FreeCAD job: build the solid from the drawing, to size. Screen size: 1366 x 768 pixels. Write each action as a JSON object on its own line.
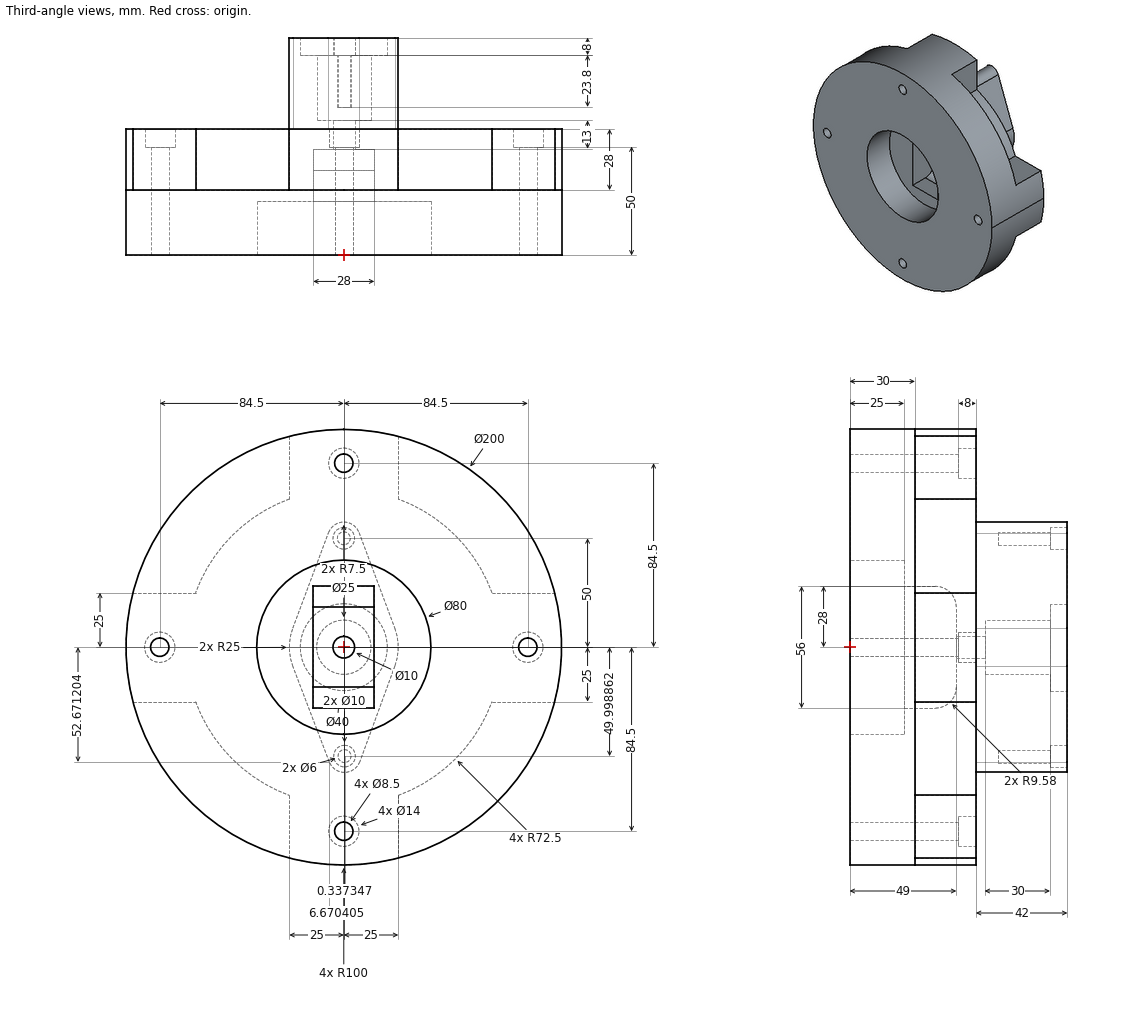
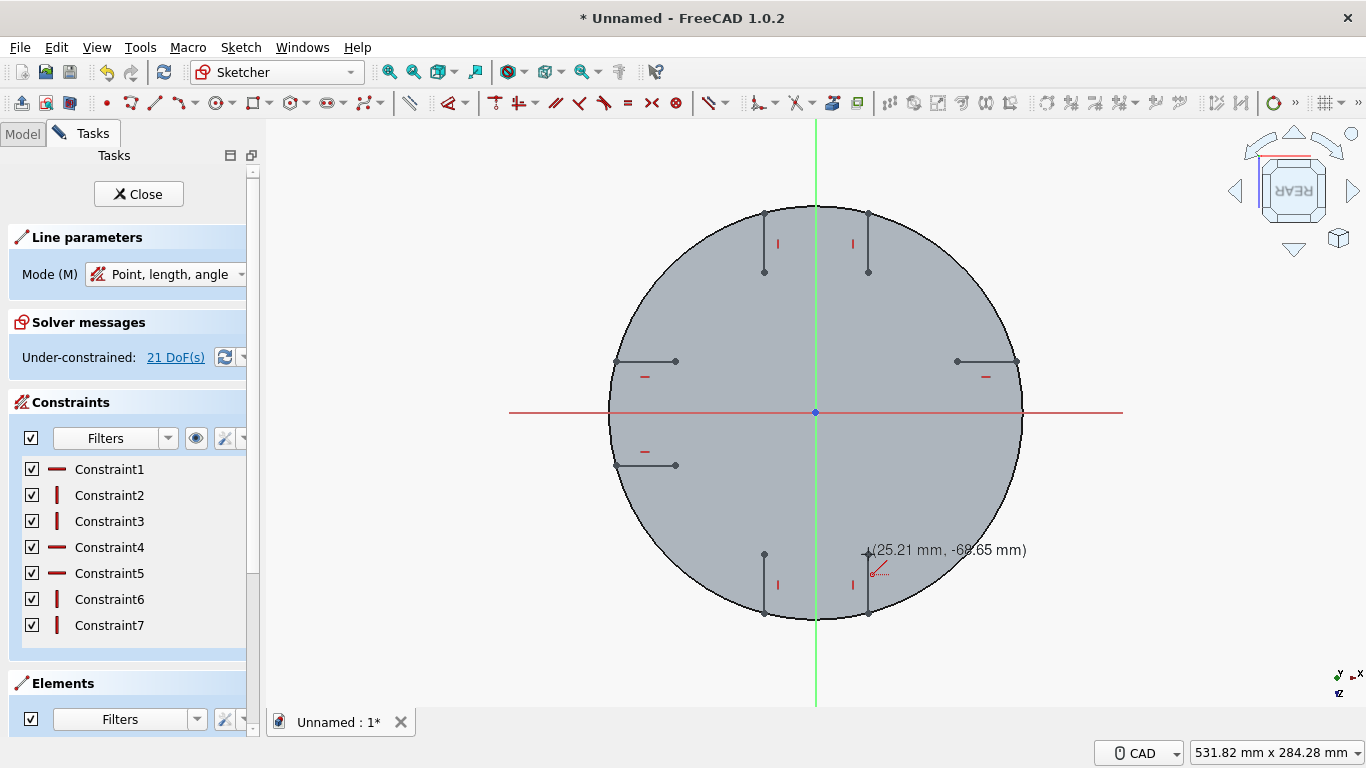
{"action": "left_click", "coordinate": [957, 465]}
{"action": "left_click", "coordinate": [1016, 465]}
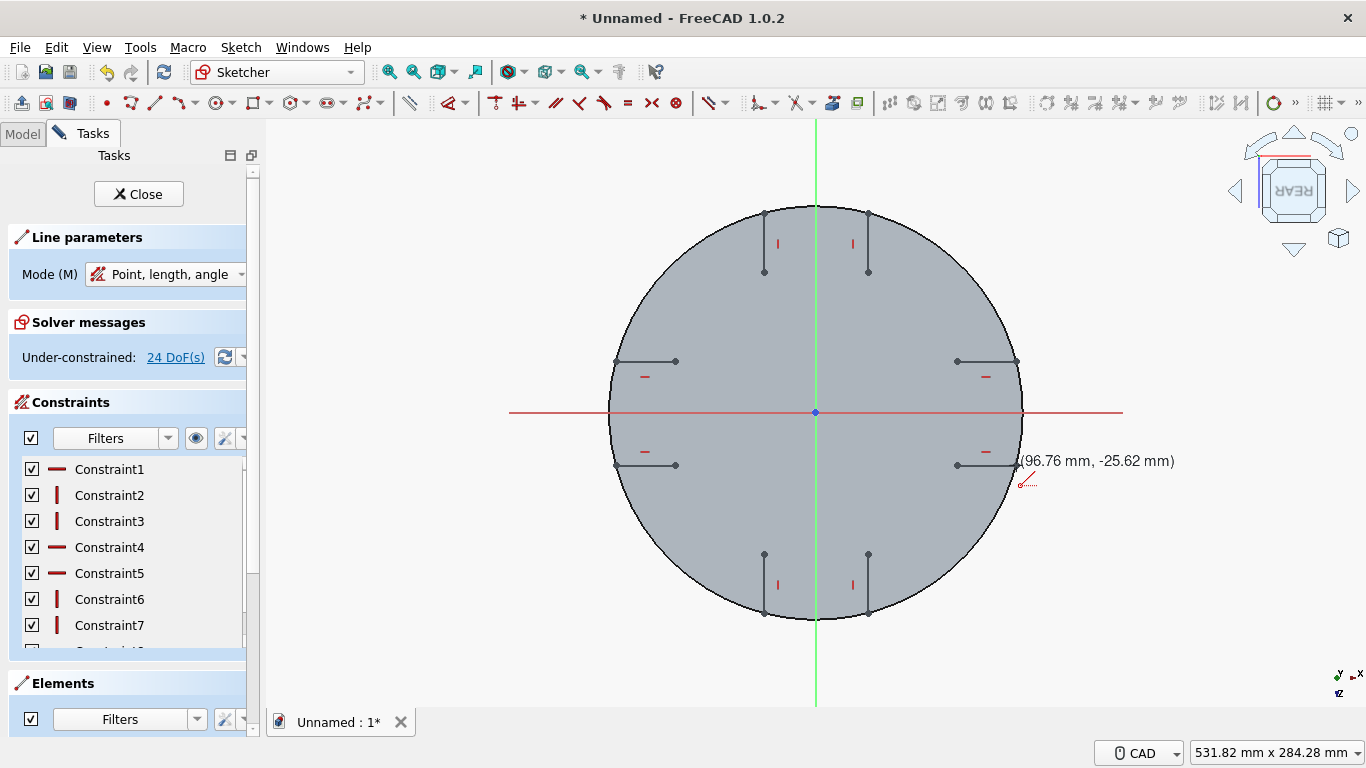
{"action": "left_click", "coordinate": [180, 104]}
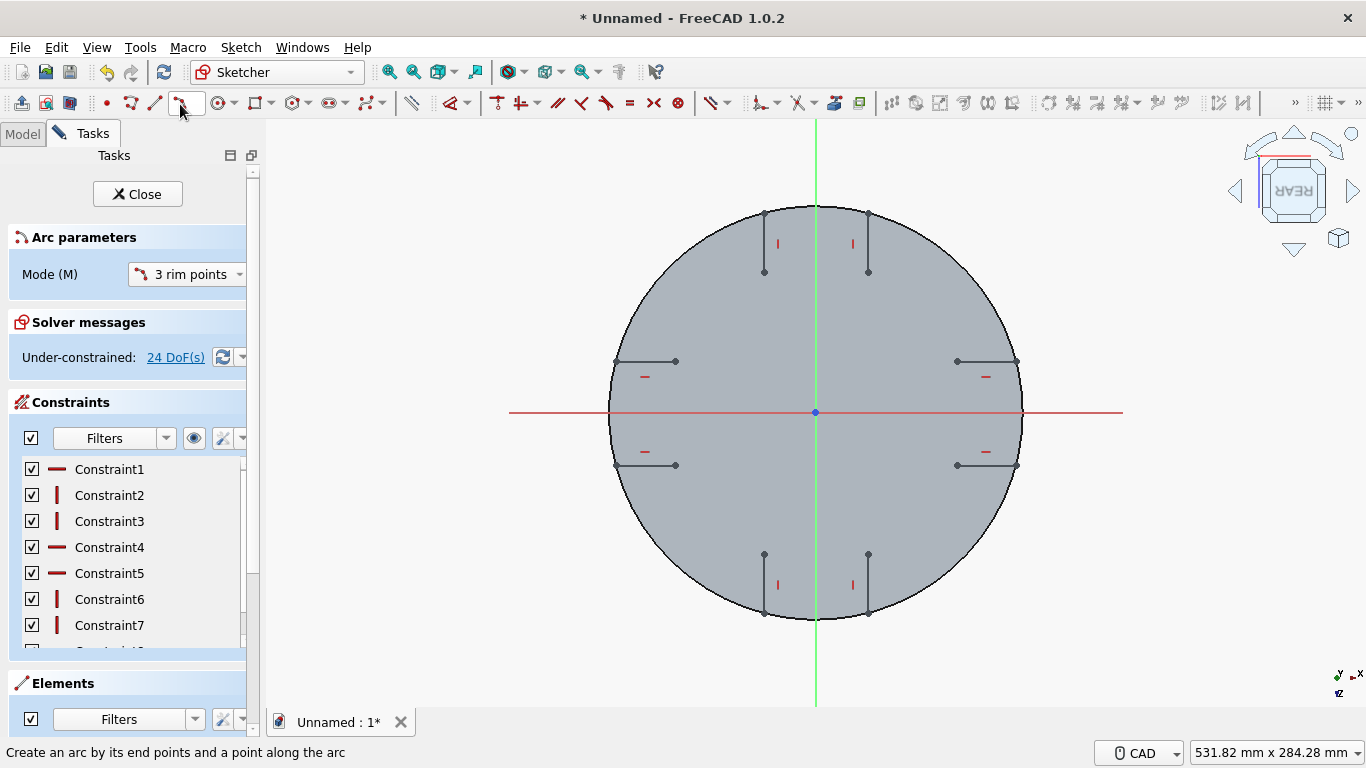
{"action": "left_click", "coordinate": [957, 362]}
{"action": "left_click", "coordinate": [868, 273]}
{"action": "left_click", "coordinate": [922, 307]}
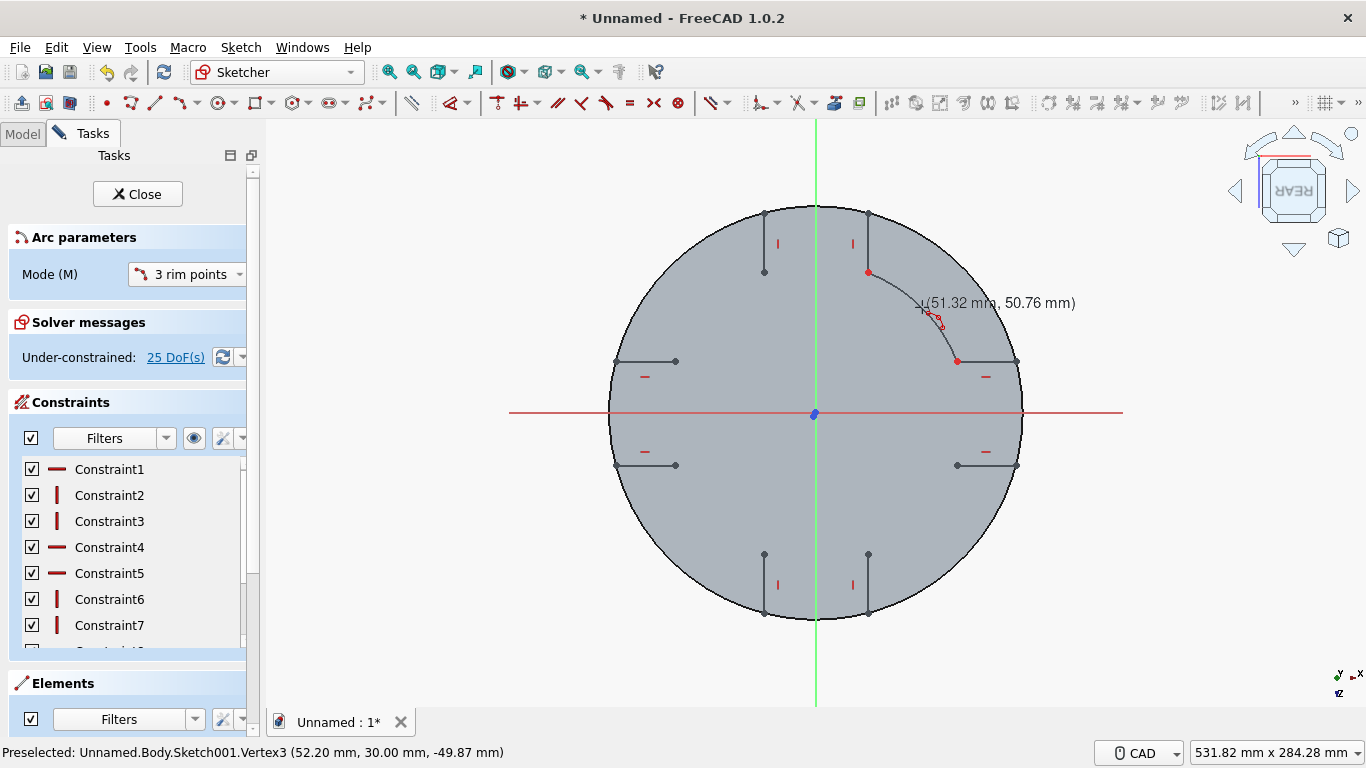
{"action": "left_click", "coordinate": [868, 214]}
{"action": "left_click", "coordinate": [764, 214]}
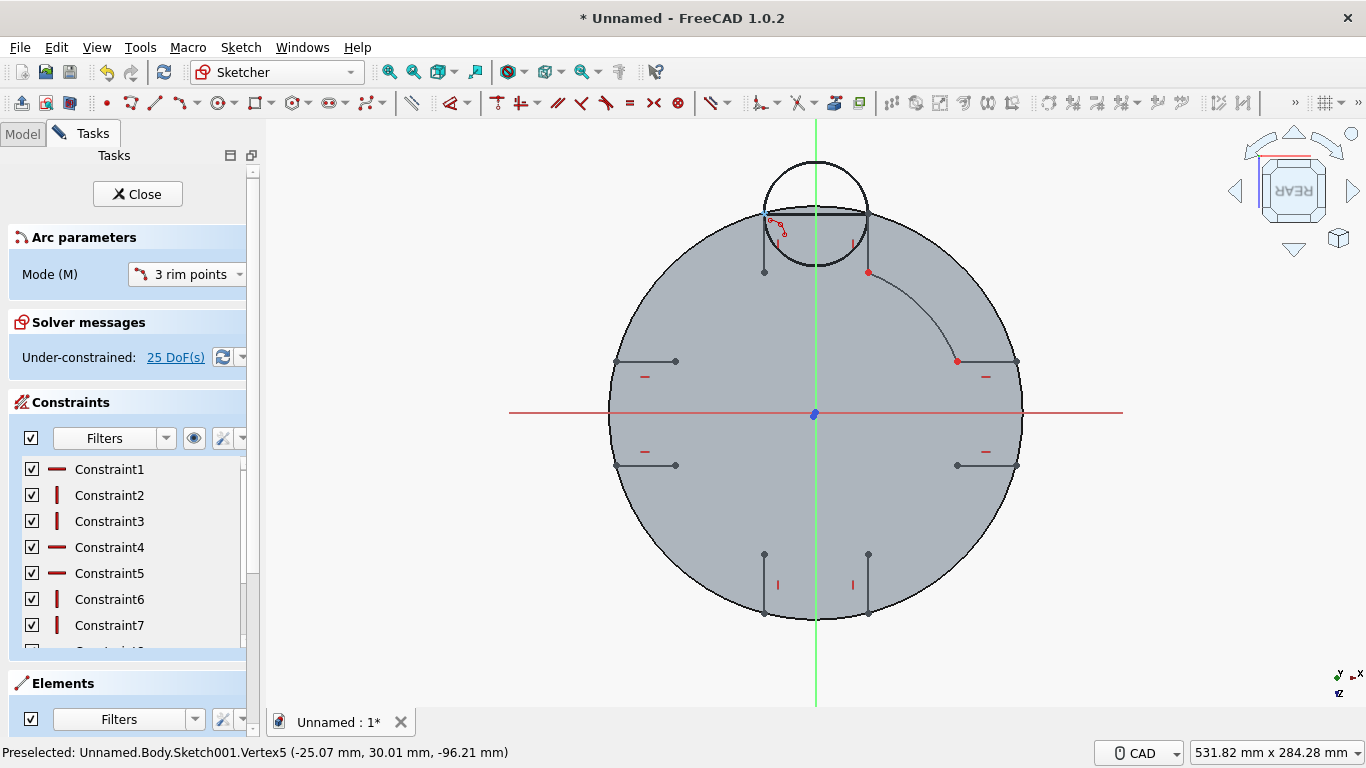
{"action": "scroll", "coordinate": [826, 206], "scroll_direction": "up", "scroll_amount": 5}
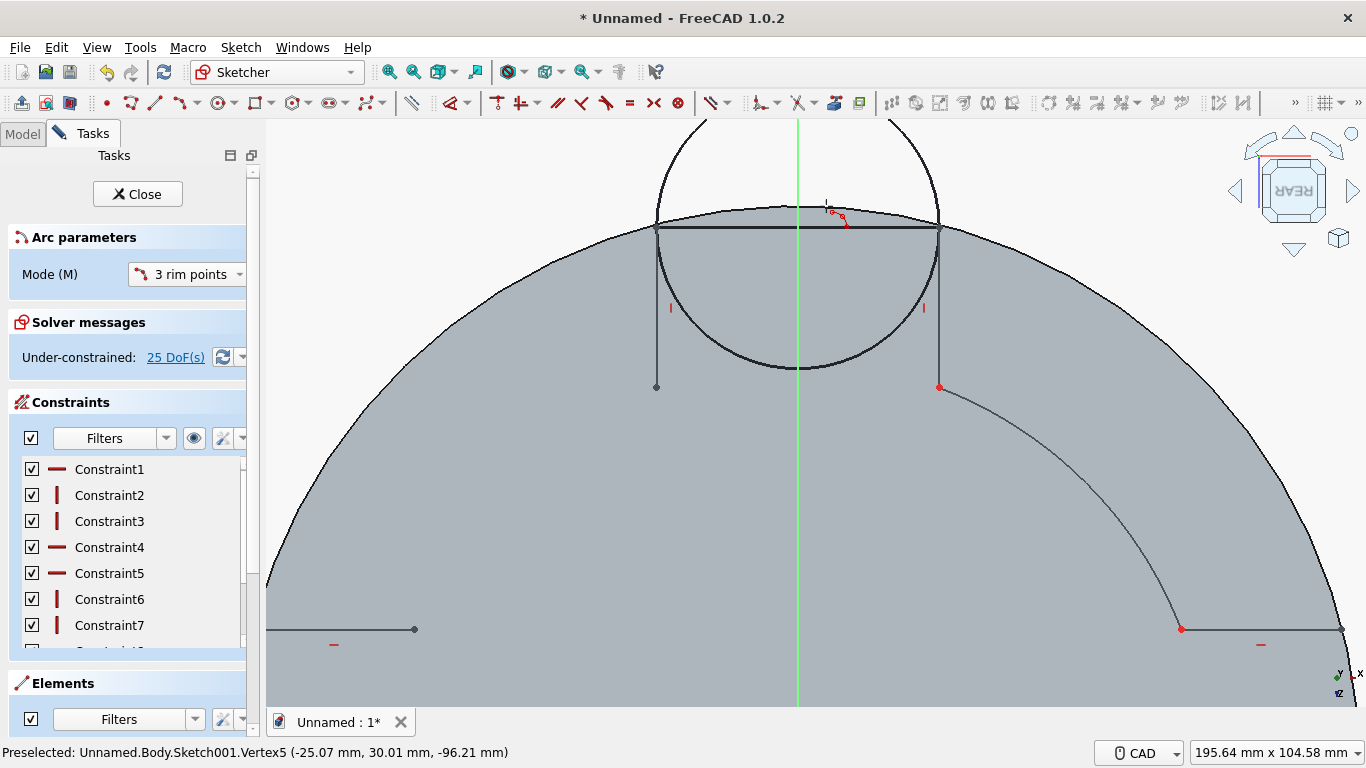
{"action": "left_click", "coordinate": [826, 207]}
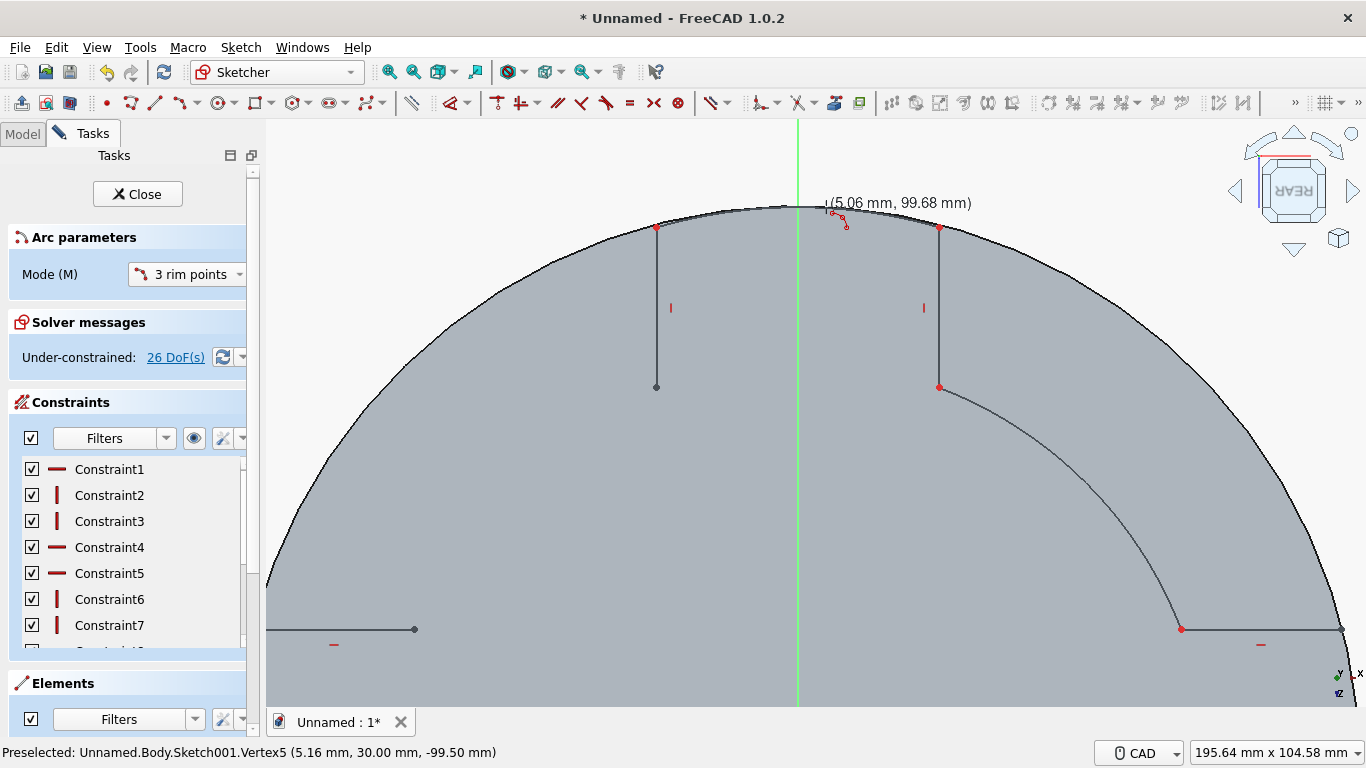
{"action": "left_click", "coordinate": [657, 388]}
{"action": "left_click", "coordinate": [415, 630]}
{"action": "left_click", "coordinate": [509, 480]}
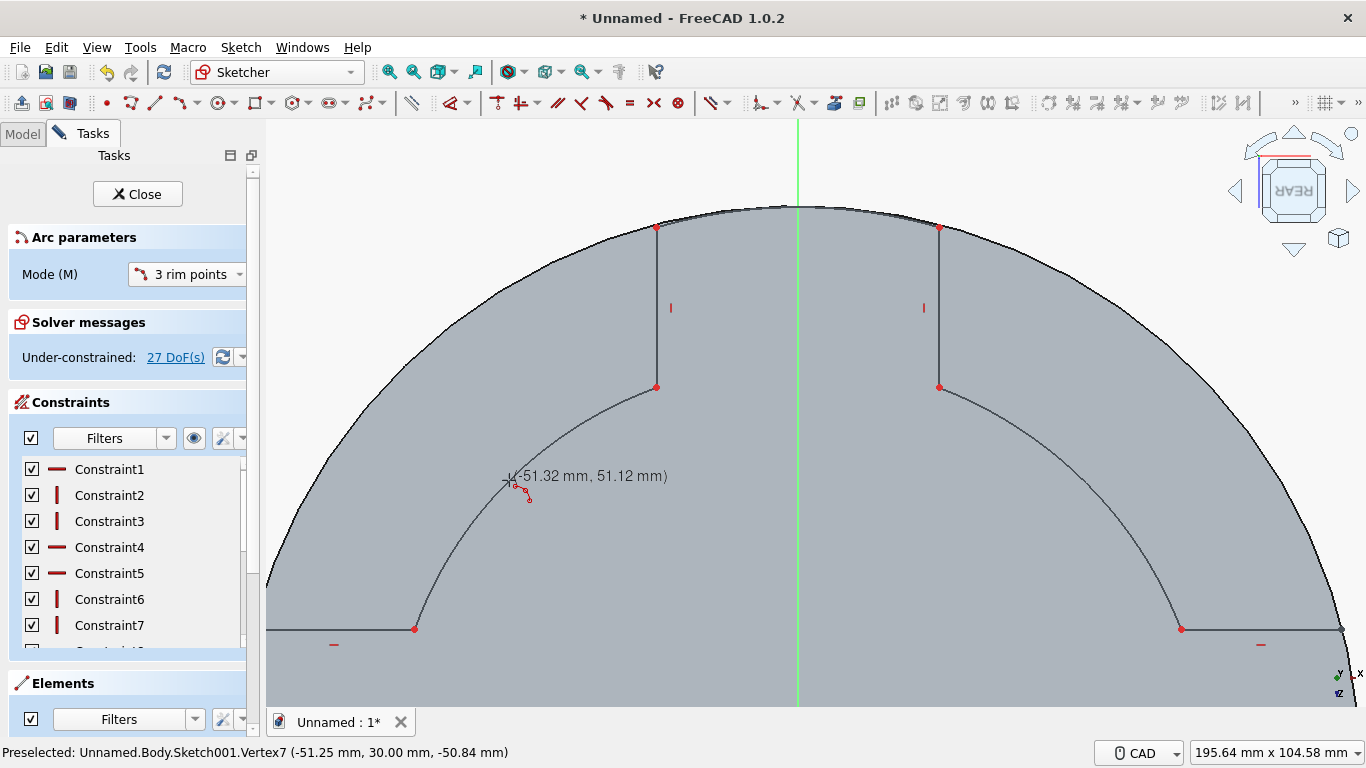
{"action": "scroll", "coordinate": [718, 206], "scroll_direction": "down", "scroll_amount": 5}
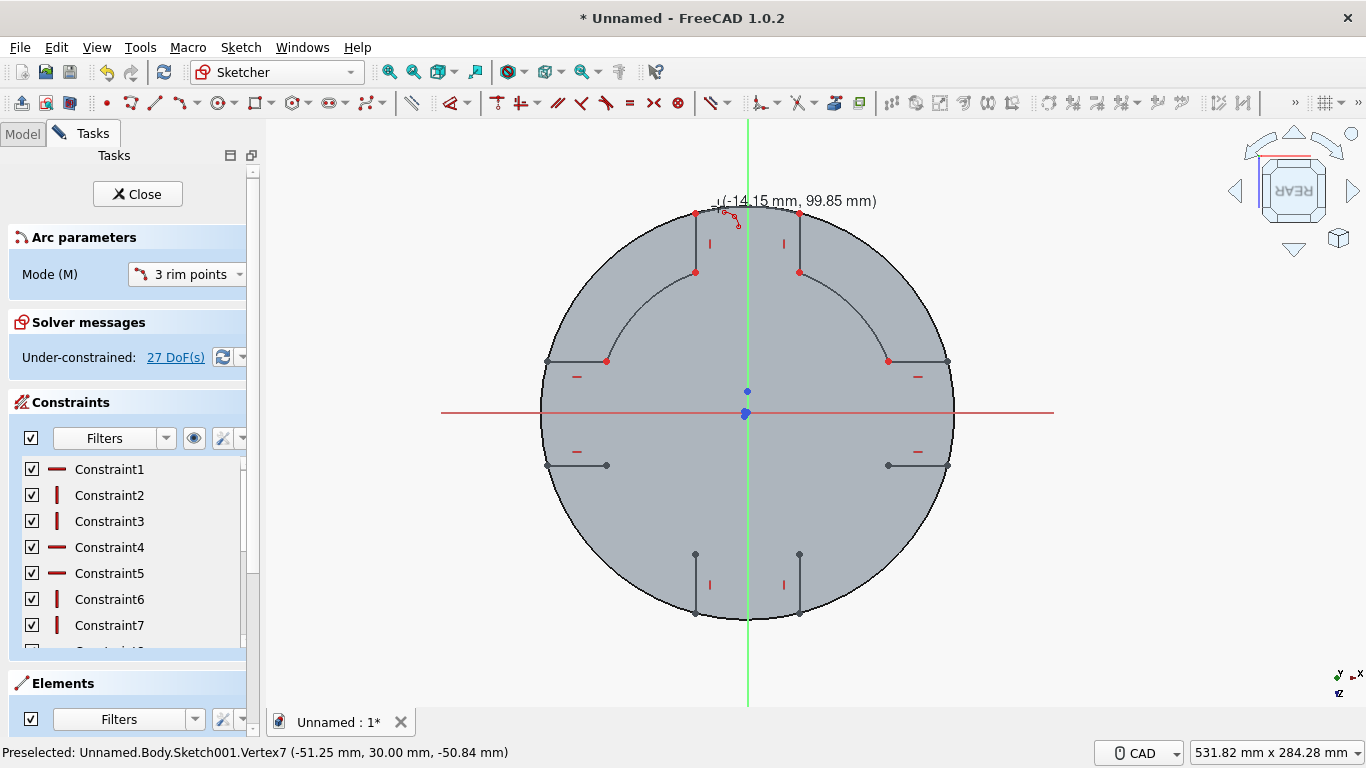
{"action": "left_click", "coordinate": [548, 362]}
{"action": "left_click", "coordinate": [548, 466]}